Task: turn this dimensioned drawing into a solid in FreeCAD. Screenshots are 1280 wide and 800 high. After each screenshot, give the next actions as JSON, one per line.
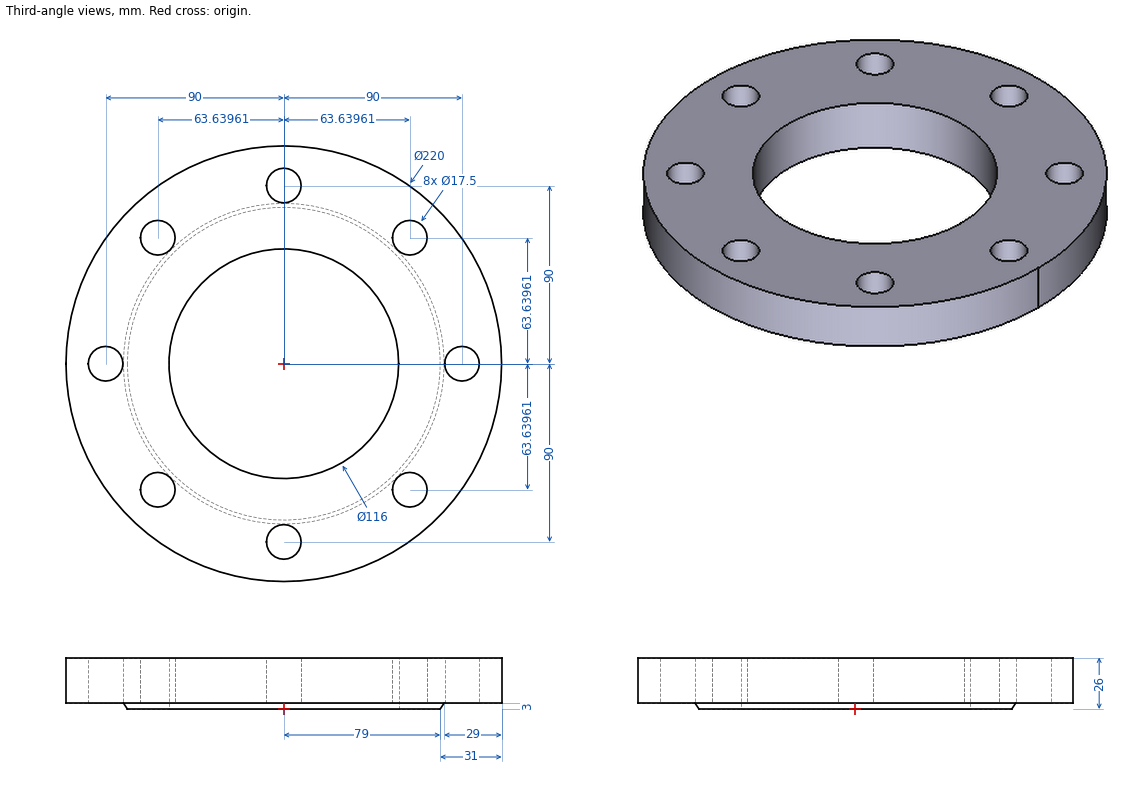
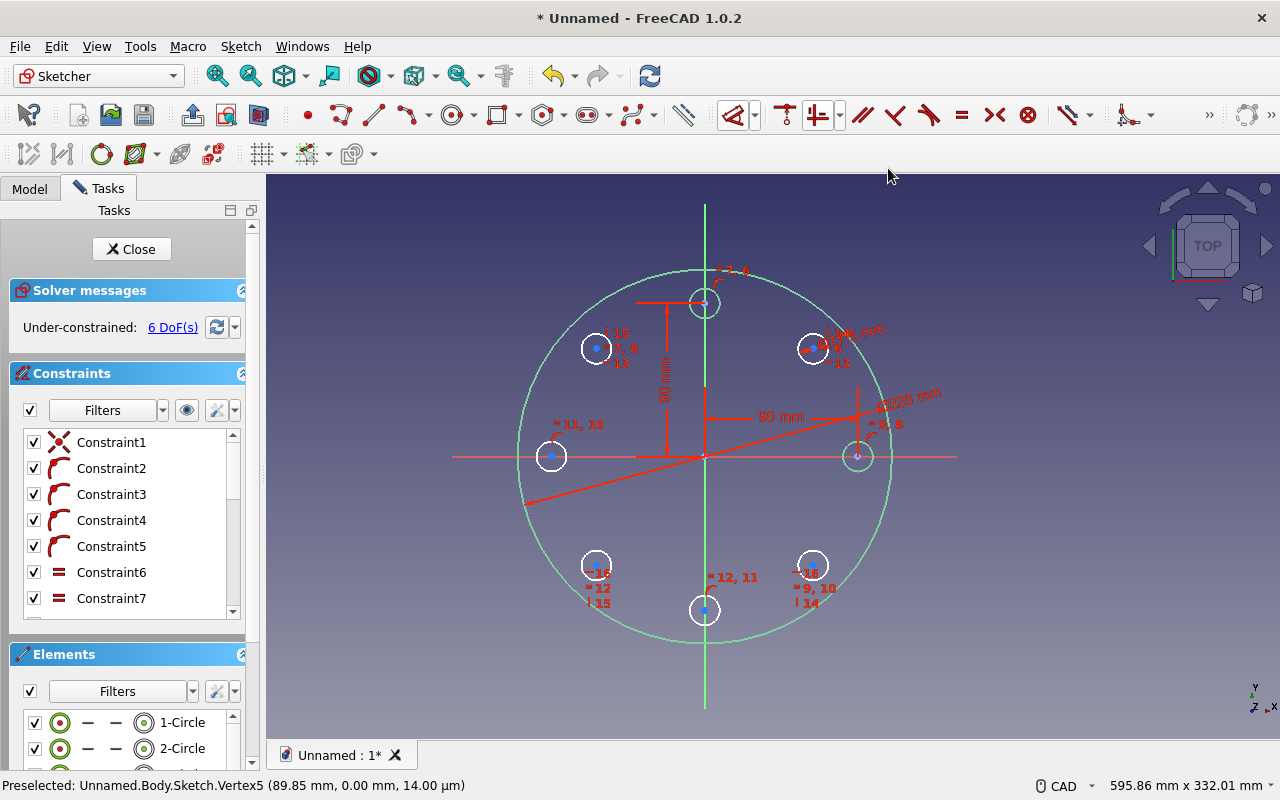
{"action": "left_click", "coordinate": [551, 457]}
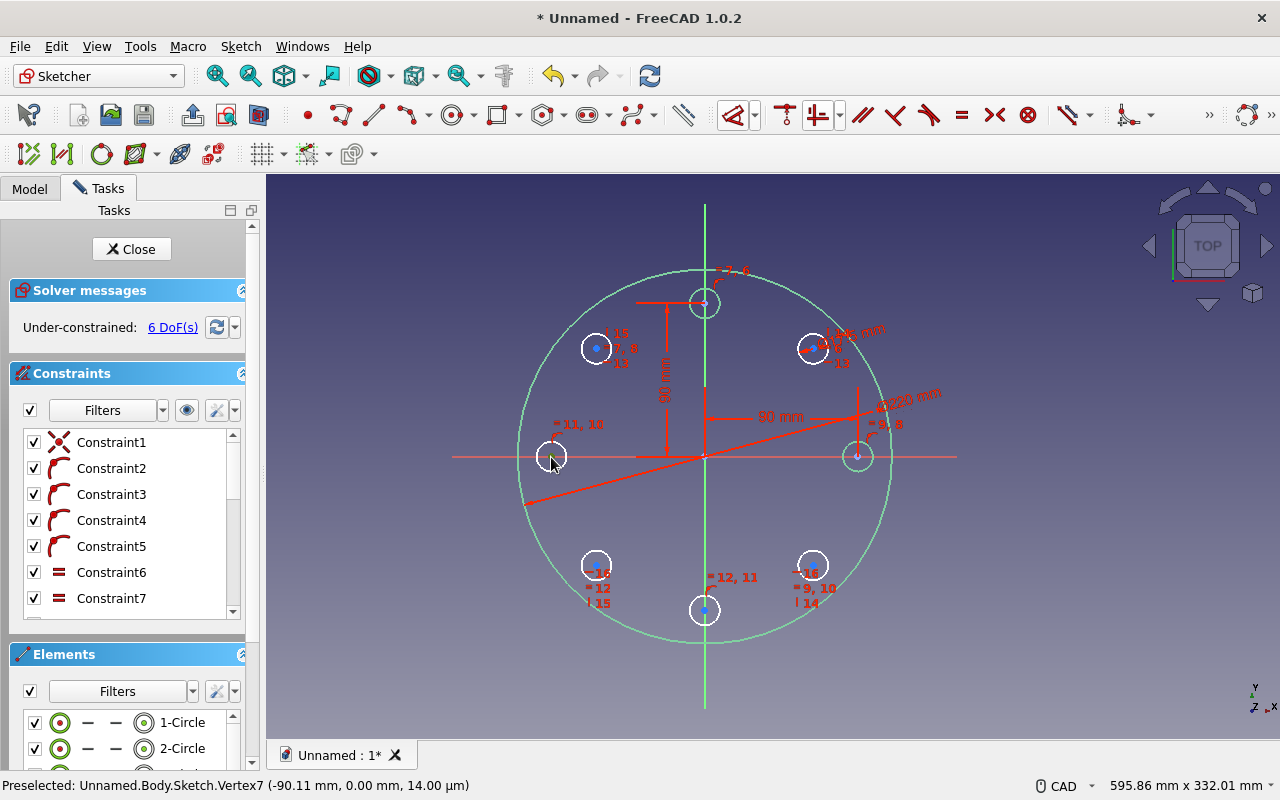
{"action": "key", "text": "l"}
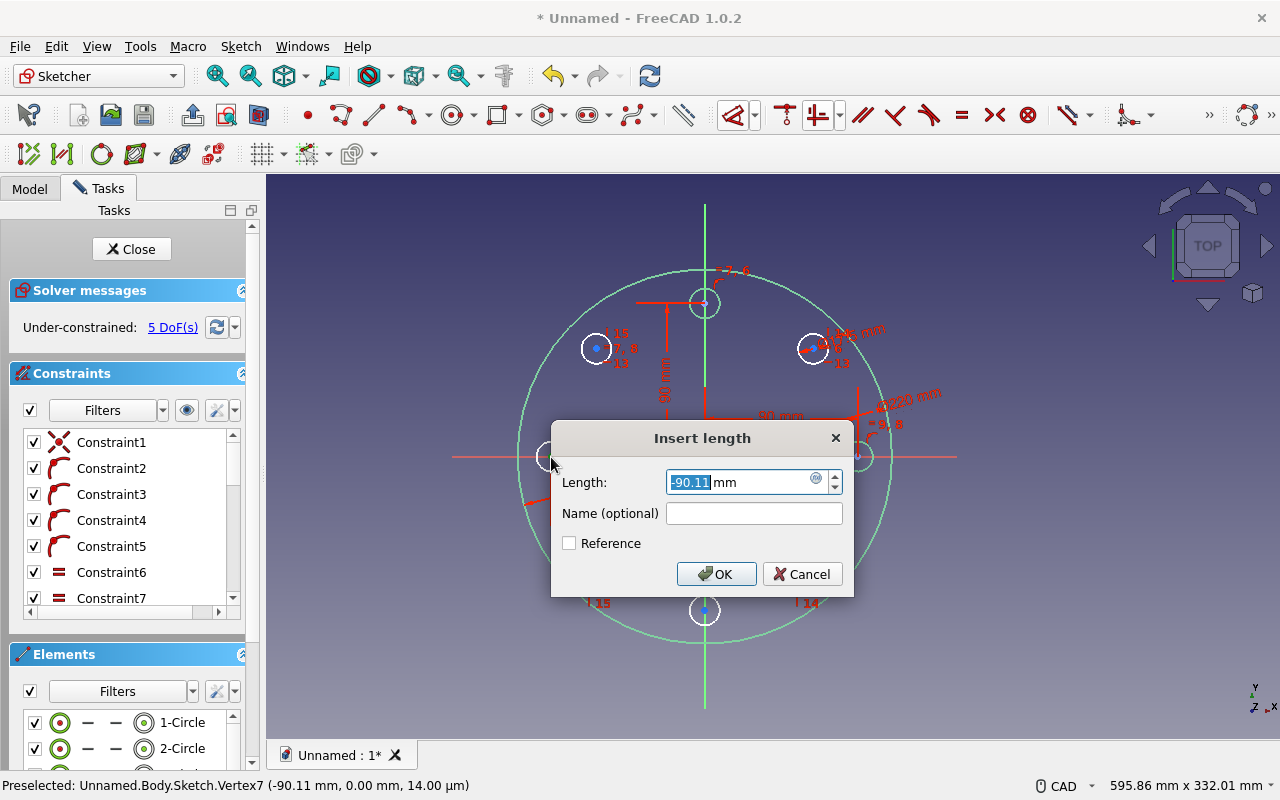
{"action": "type", "text": "-90"}
{"action": "key", "text": "Return"}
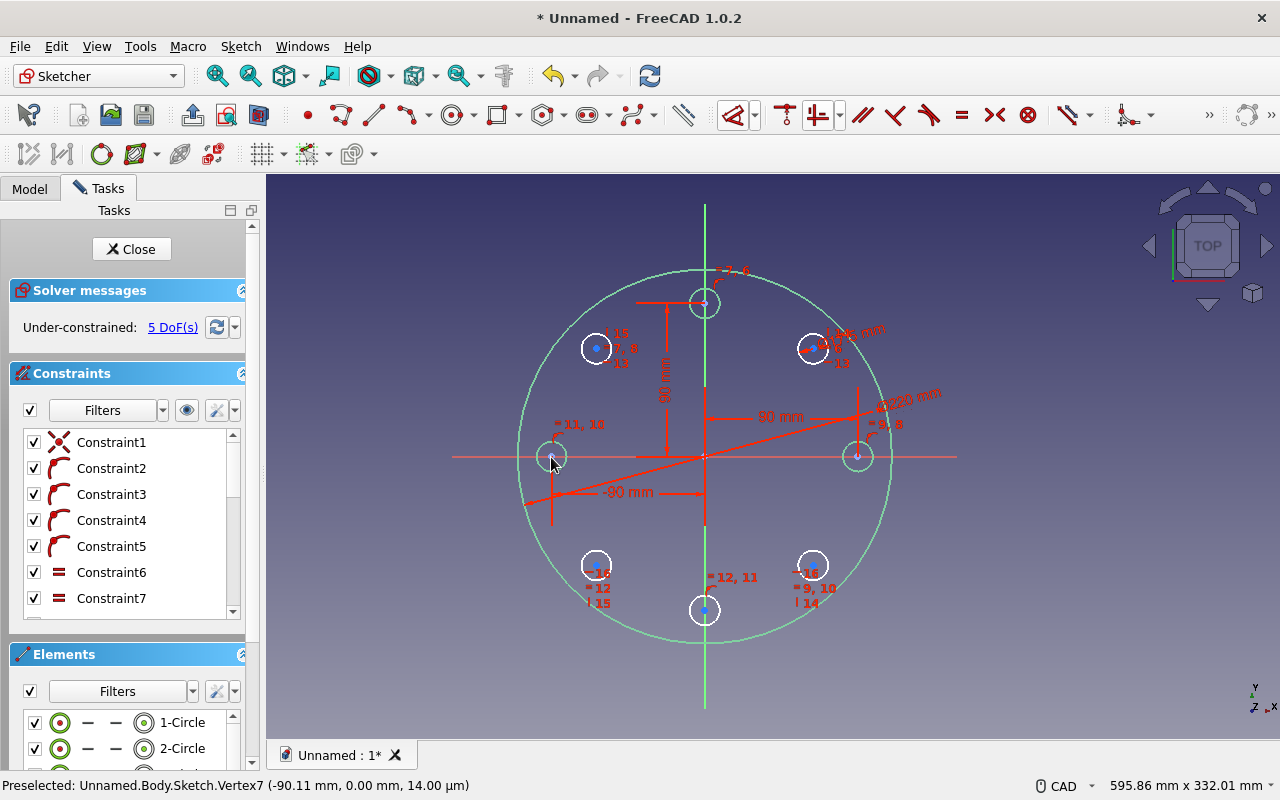
{"action": "left_click", "coordinate": [705, 610]}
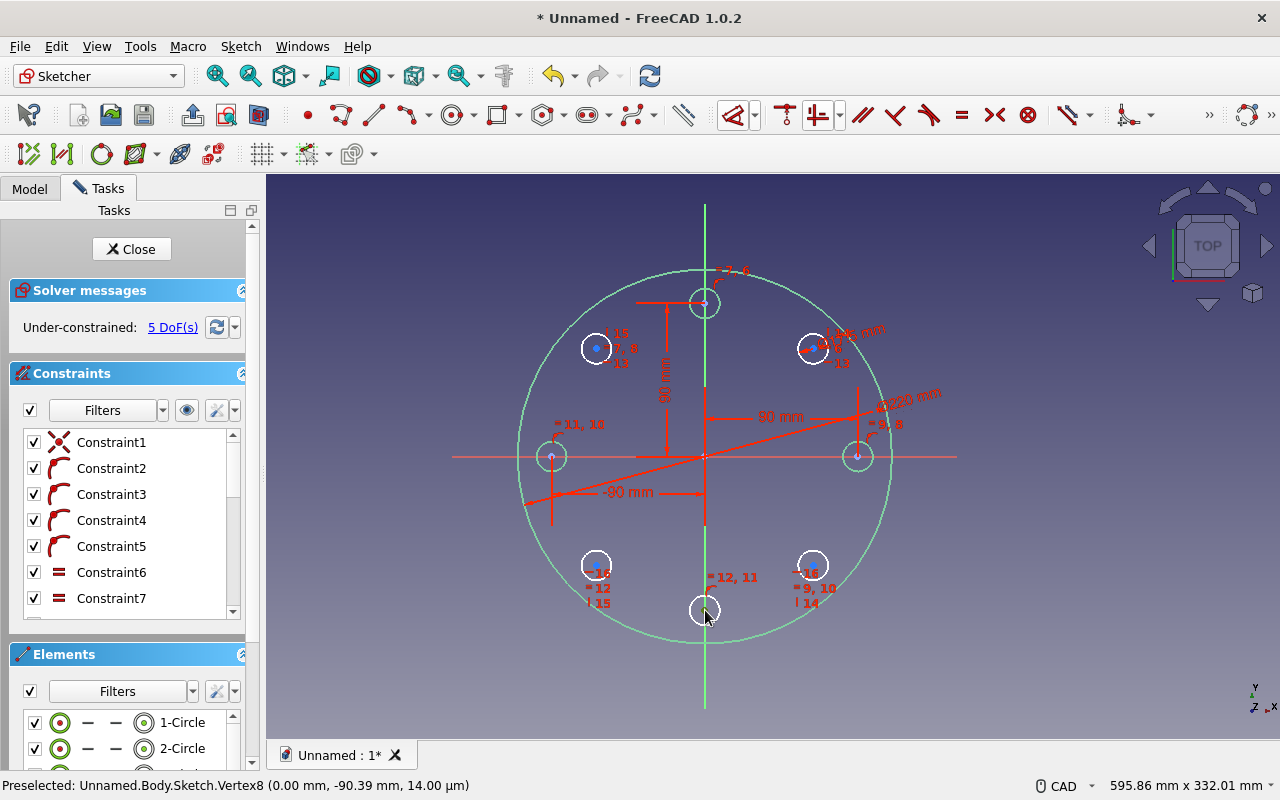
{"action": "left_click", "coordinate": [754, 116]}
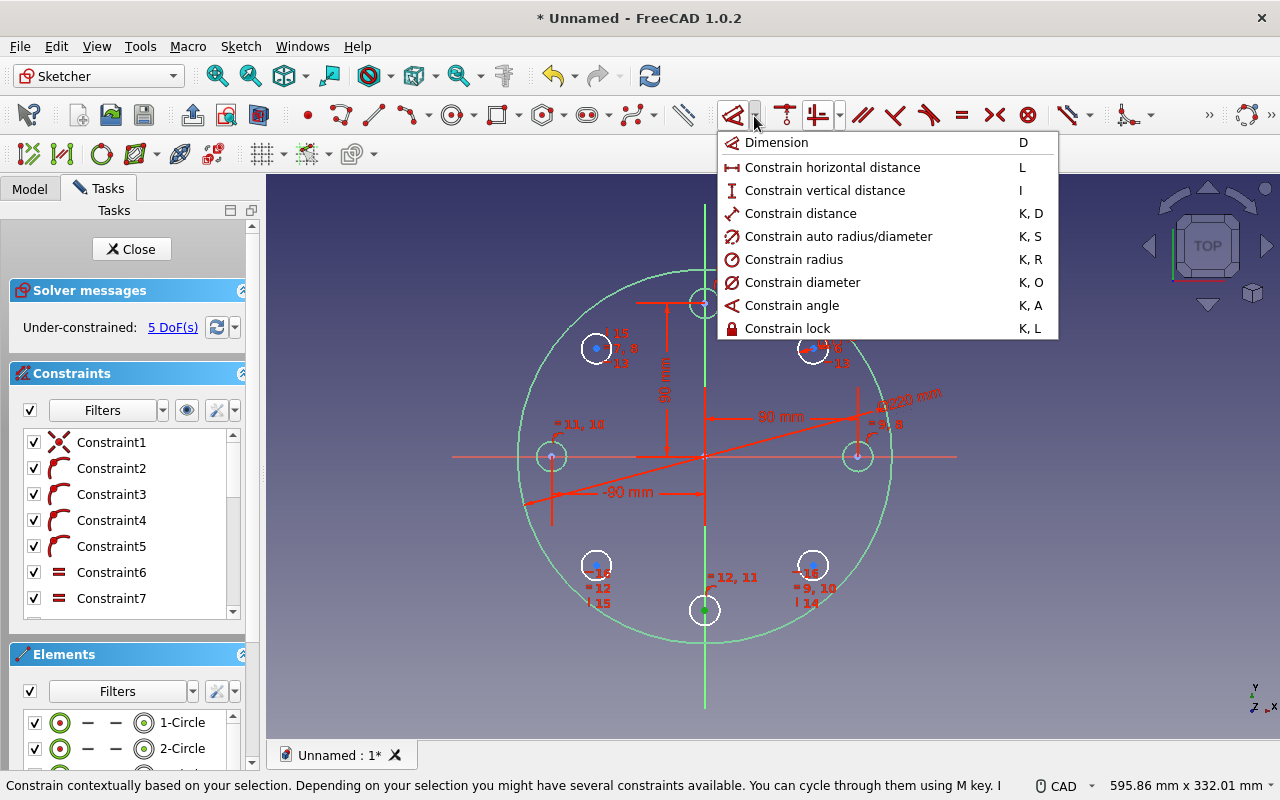
{"action": "left_click", "coordinate": [888, 190]}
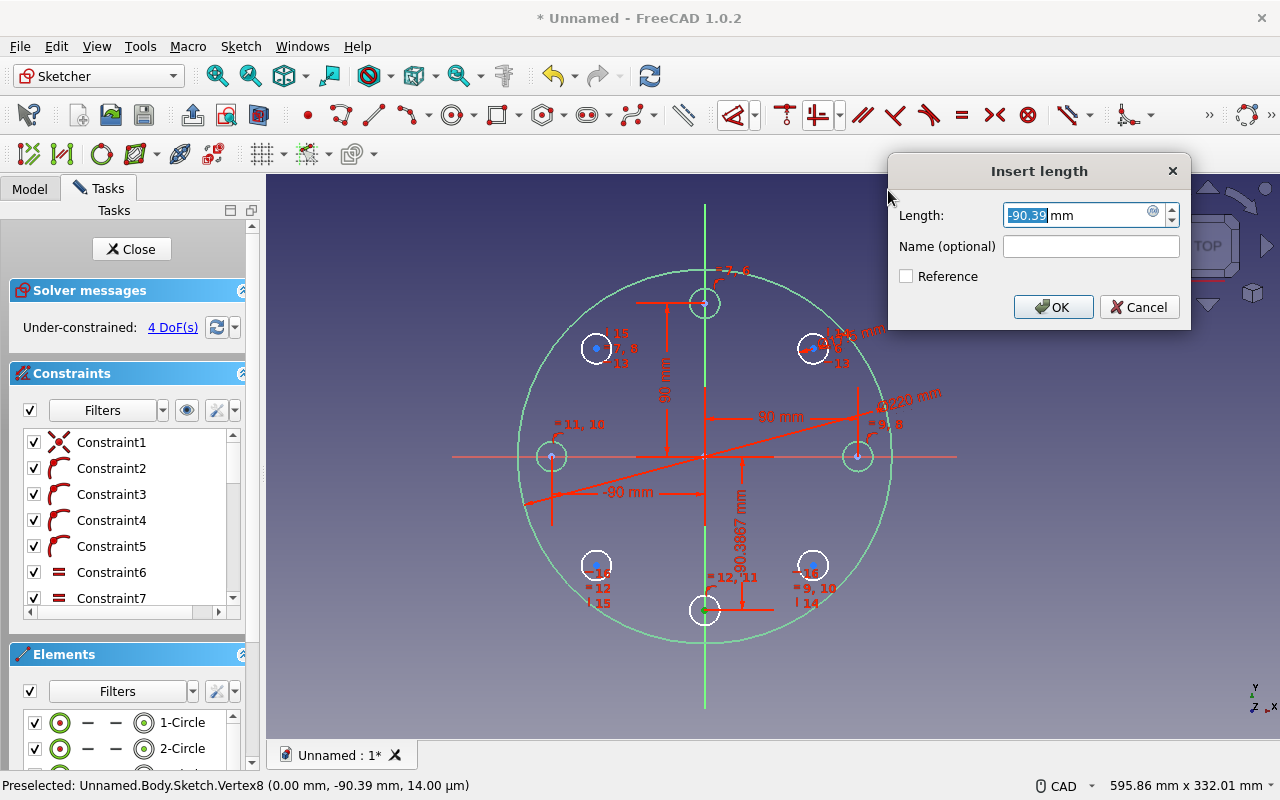
{"action": "type", "text": "-90"}
{"action": "key", "text": "Return"}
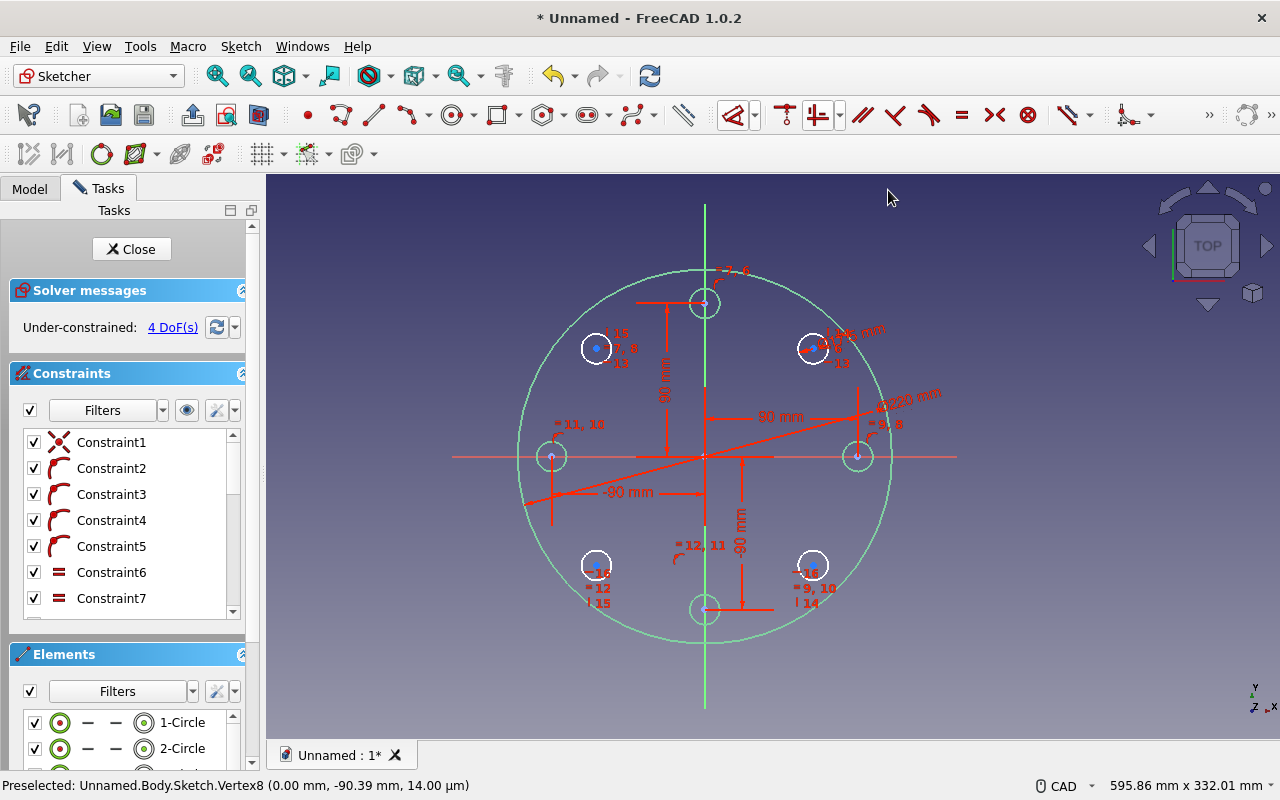
{"action": "left_click", "coordinate": [813, 349]}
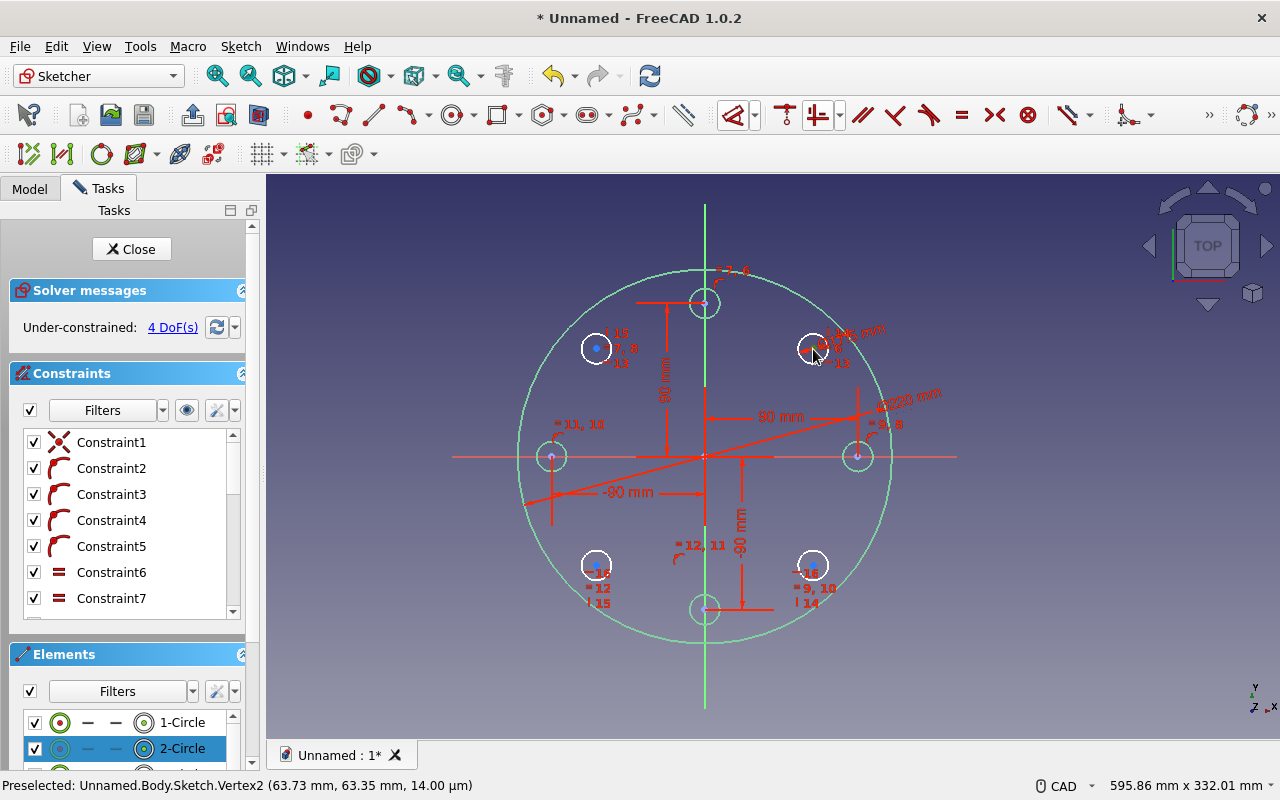
{"action": "key", "text": "l"}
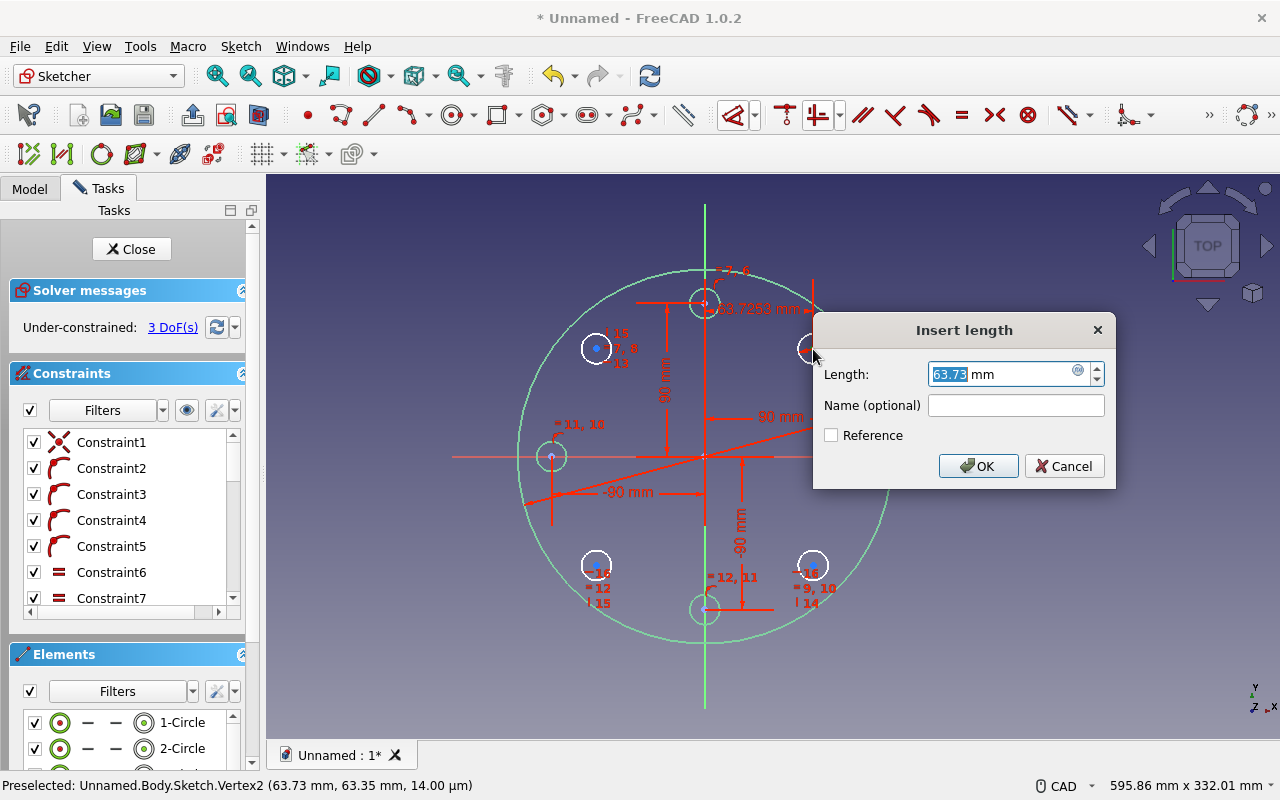
{"action": "type", "text": "63.63961"}
{"action": "key", "text": "Return"}